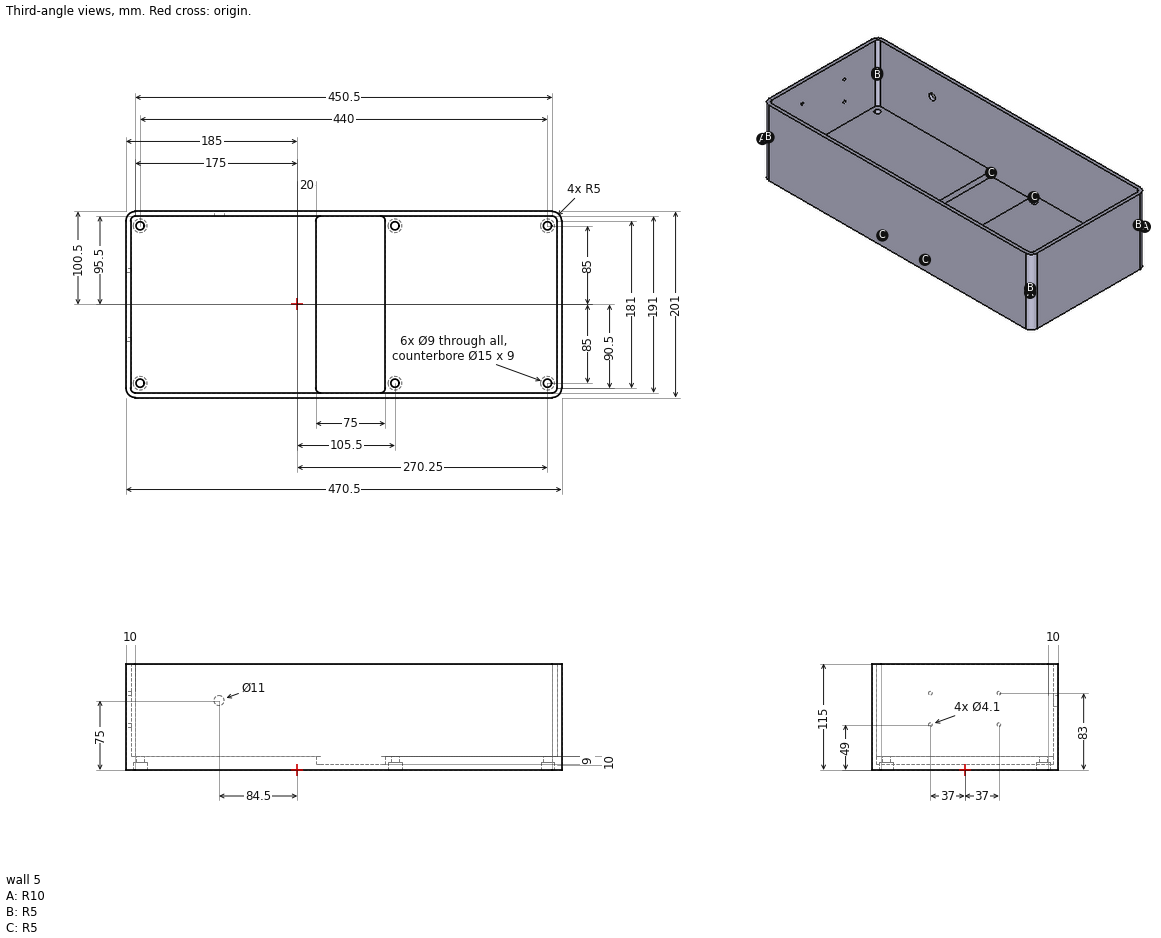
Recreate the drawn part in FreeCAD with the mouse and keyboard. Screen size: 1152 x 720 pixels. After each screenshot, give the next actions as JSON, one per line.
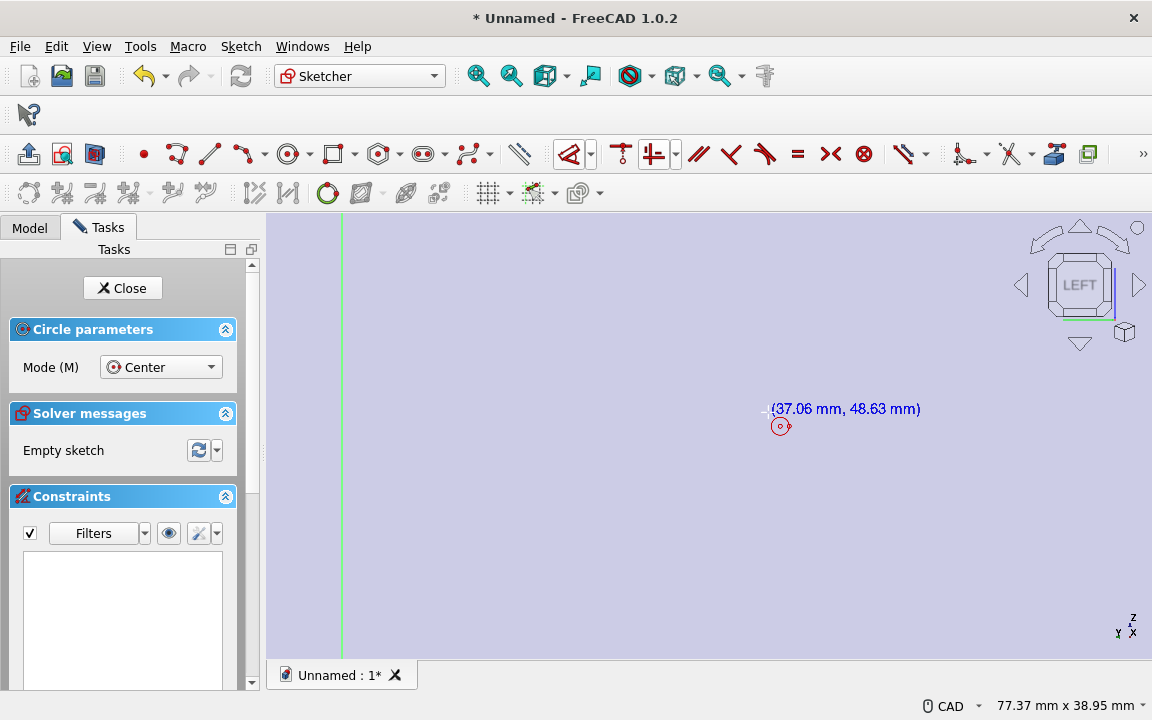
{"action": "left_click", "coordinate": [766, 410]}
{"action": "mouse_move", "coordinate": [783, 393]}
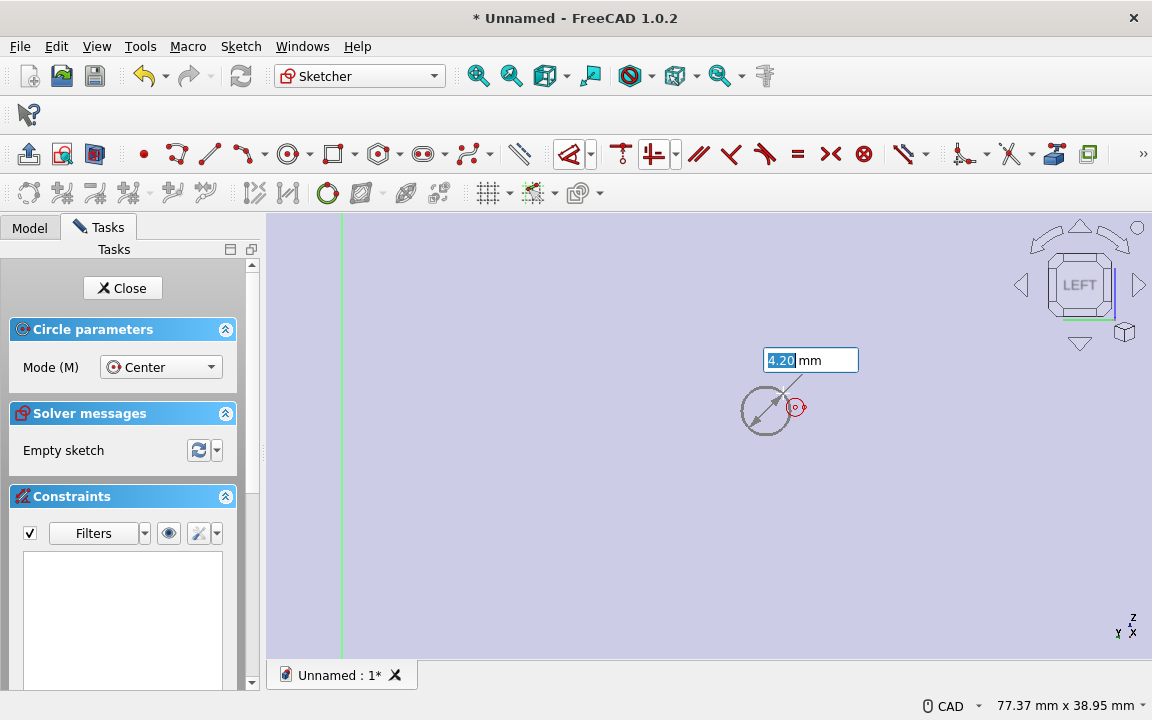
{"action": "type", "text": "4.1"}
{"action": "key", "text": "Return"}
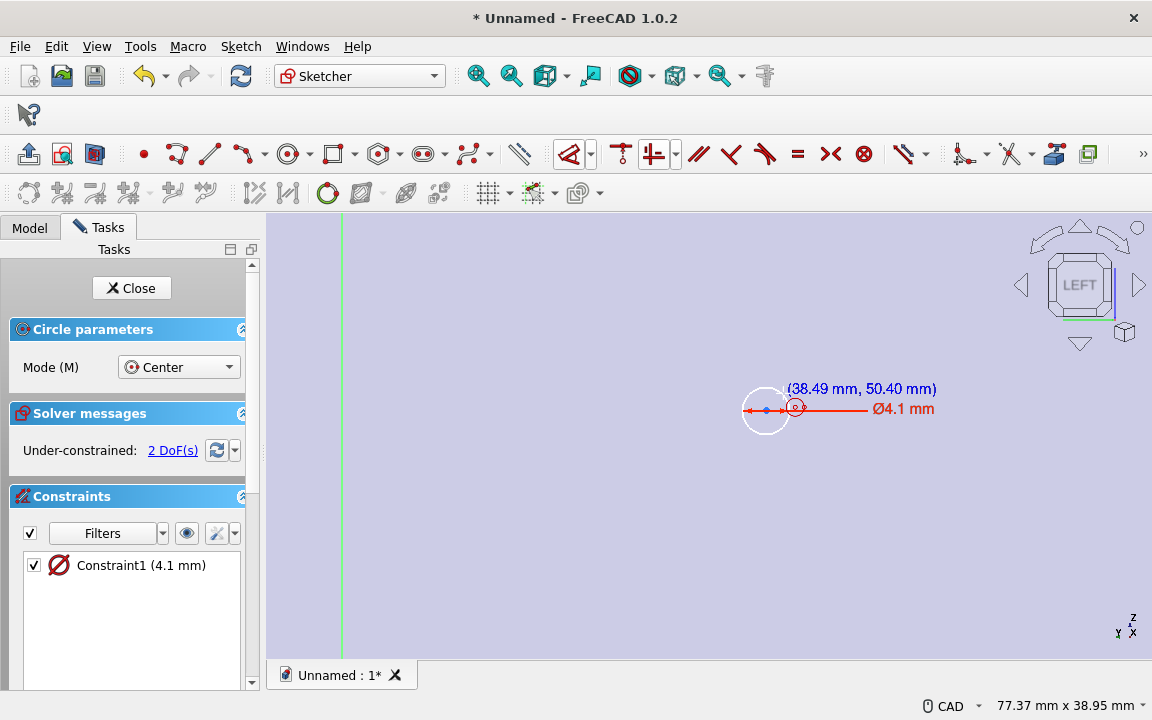
{"action": "scroll", "coordinate": [769, 415], "scroll_direction": "down", "scroll_amount": 6}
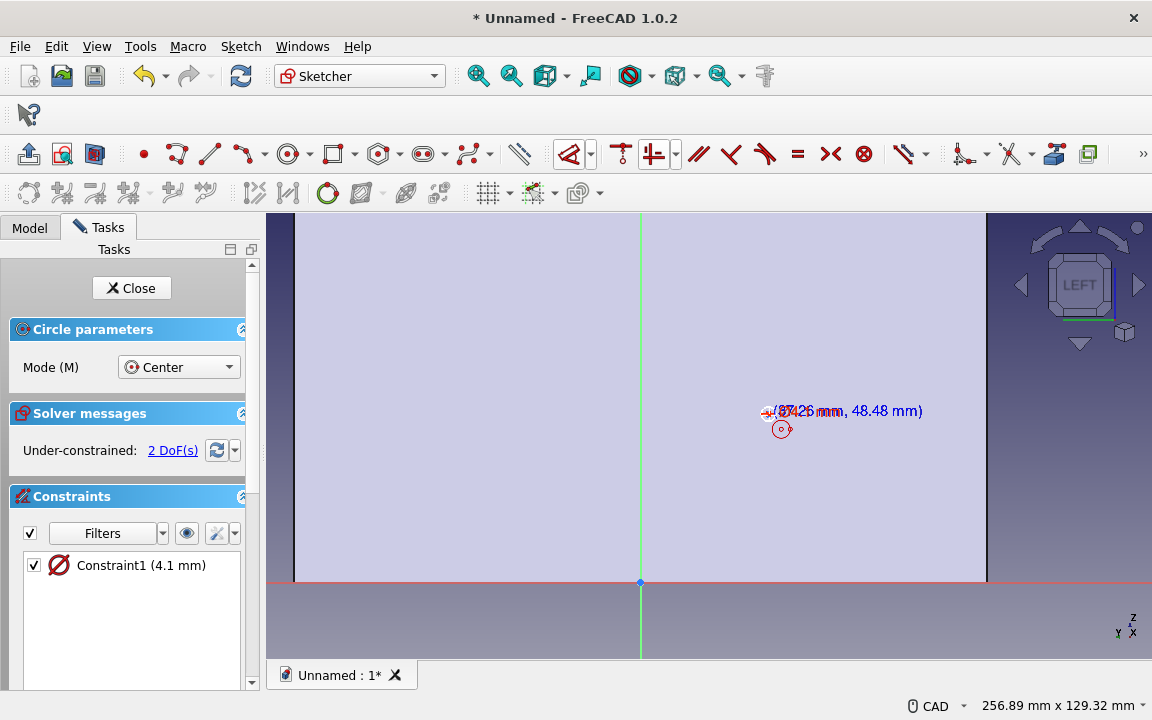
{"action": "scroll", "coordinate": [513, 414], "scroll_direction": "up", "scroll_amount": 6}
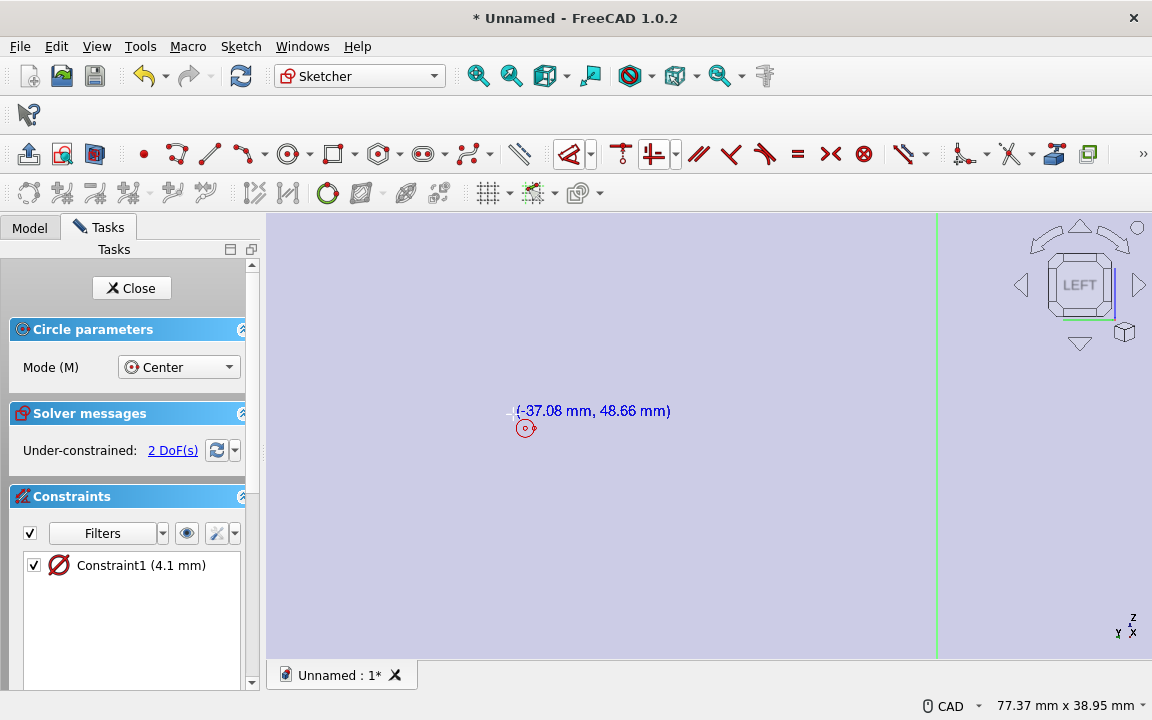
{"action": "left_click", "coordinate": [513, 412]}
{"action": "mouse_move", "coordinate": [530, 396]}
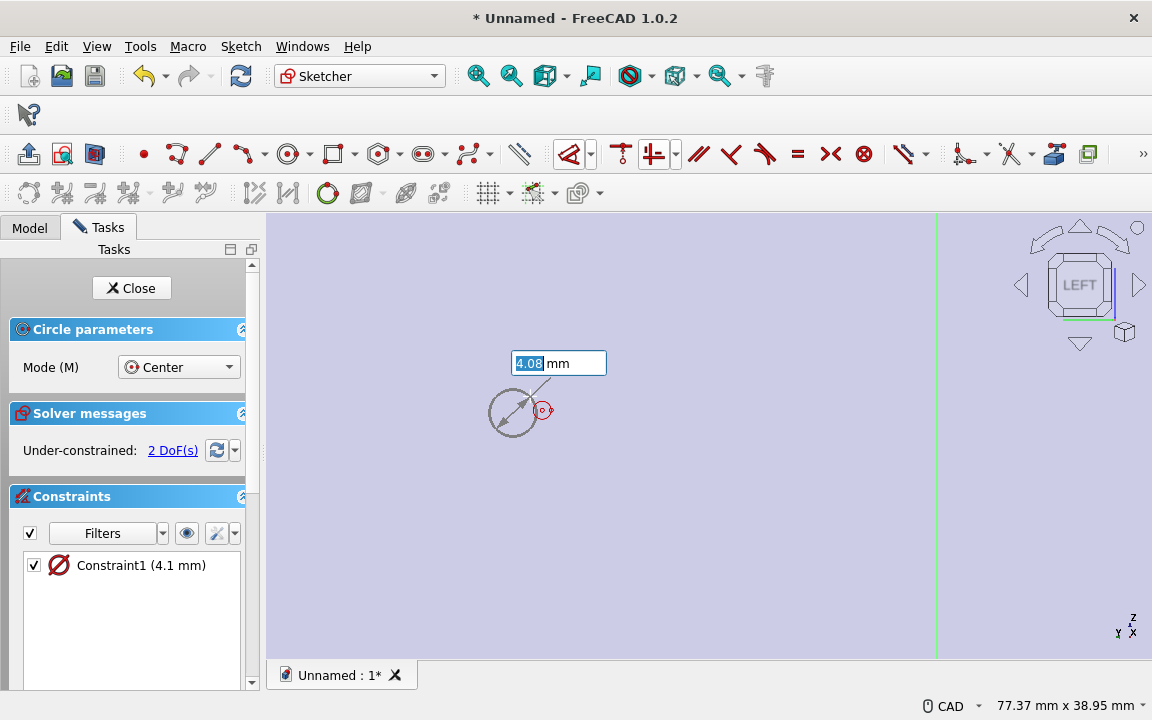
{"action": "type", "text": "4.1"}
{"action": "key", "text": "Return"}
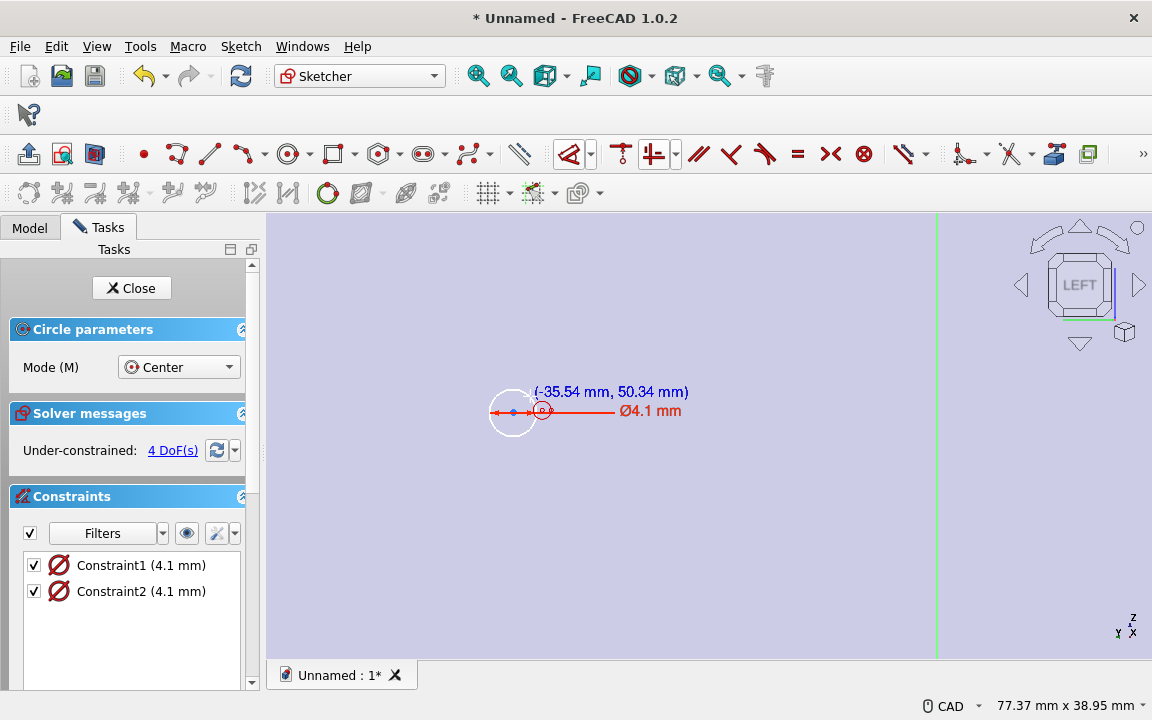
{"action": "scroll", "coordinate": [513, 414], "scroll_direction": "down", "scroll_amount": 6}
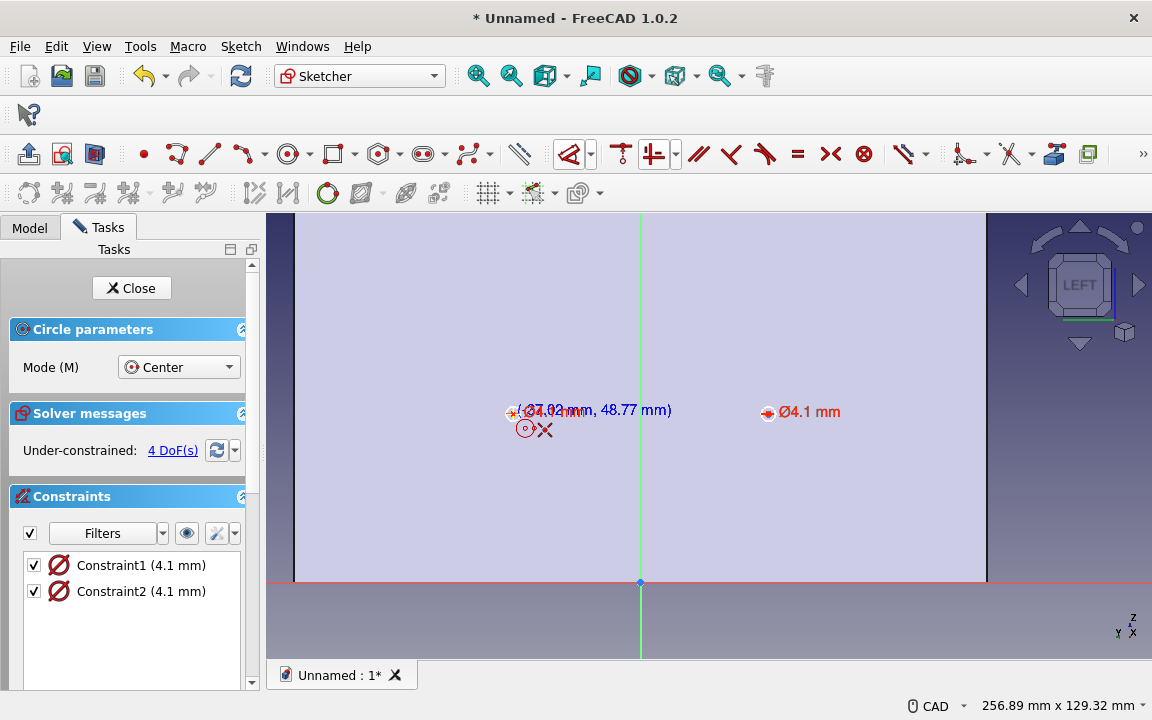
{"action": "scroll", "coordinate": [513, 297], "scroll_direction": "up", "scroll_amount": 6}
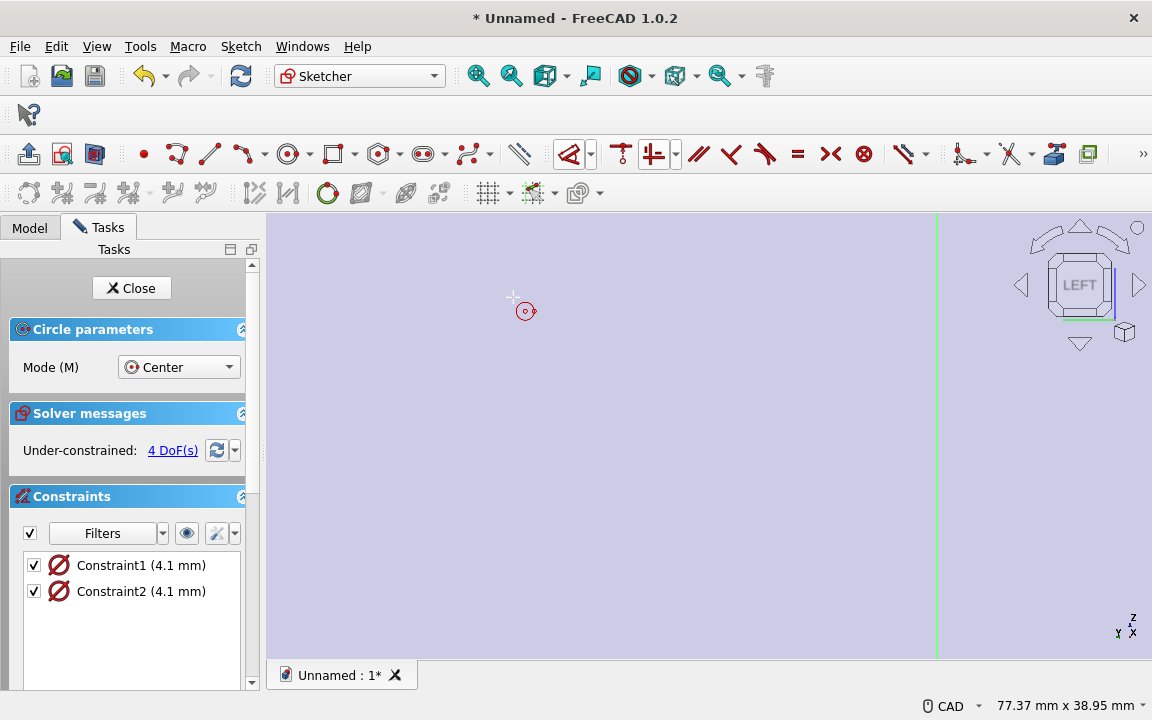
{"action": "left_click", "coordinate": [513, 295]}
{"action": "mouse_move", "coordinate": [530, 279]}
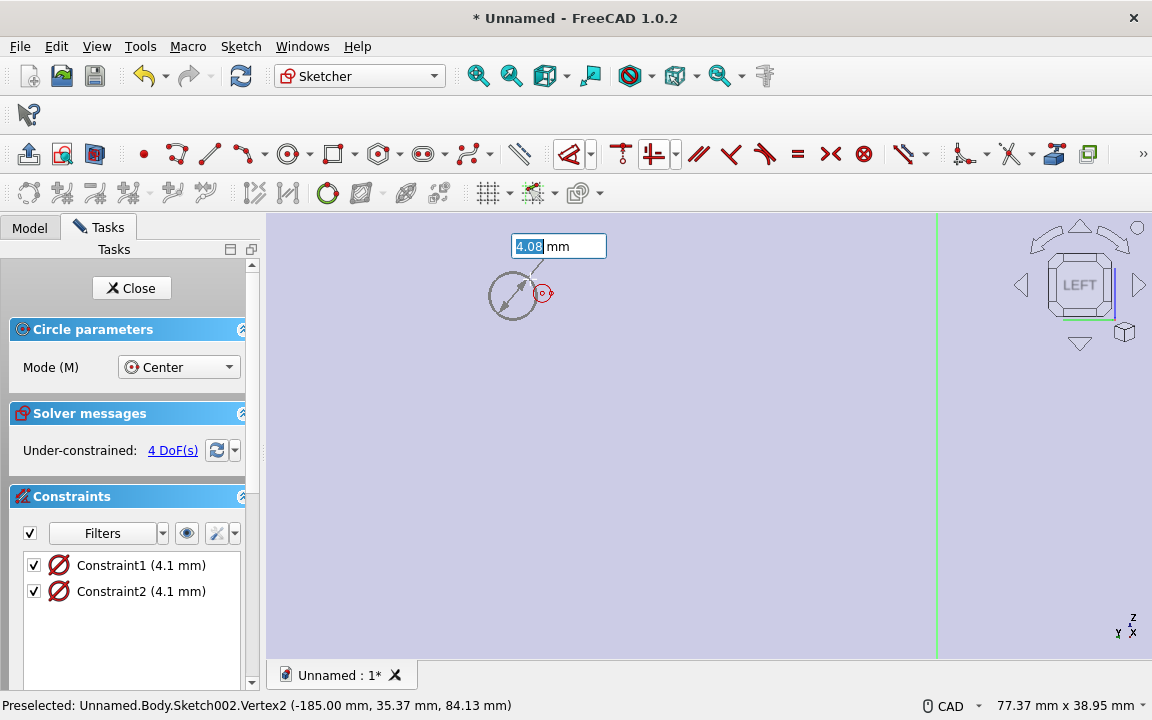
{"action": "type", "text": "4.1"}
{"action": "key", "text": "Return"}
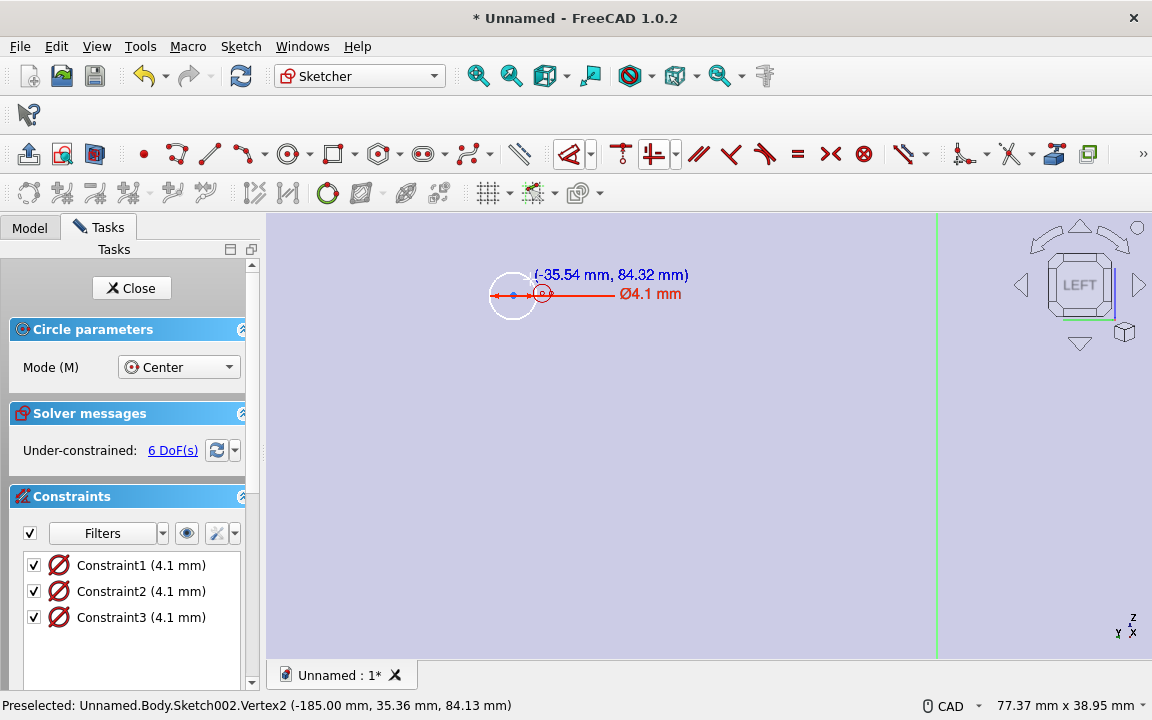
{"action": "scroll", "coordinate": [513, 297], "scroll_direction": "down", "scroll_amount": 6}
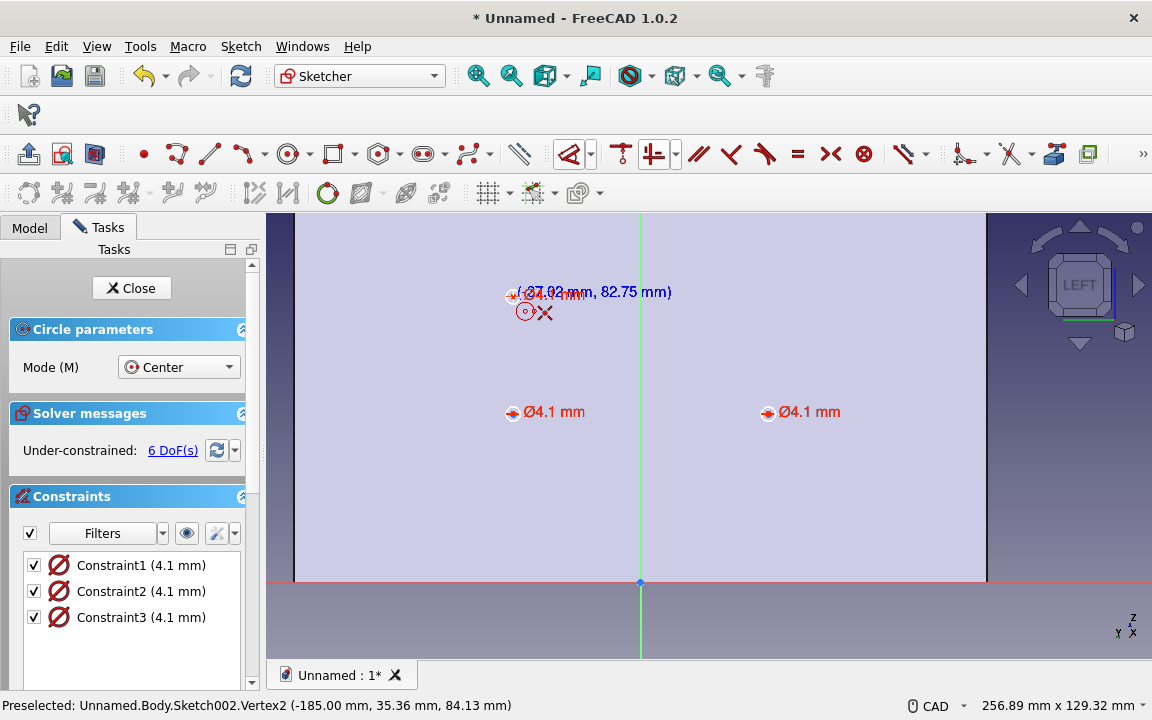
{"action": "scroll", "coordinate": [768, 297], "scroll_direction": "up", "scroll_amount": 6}